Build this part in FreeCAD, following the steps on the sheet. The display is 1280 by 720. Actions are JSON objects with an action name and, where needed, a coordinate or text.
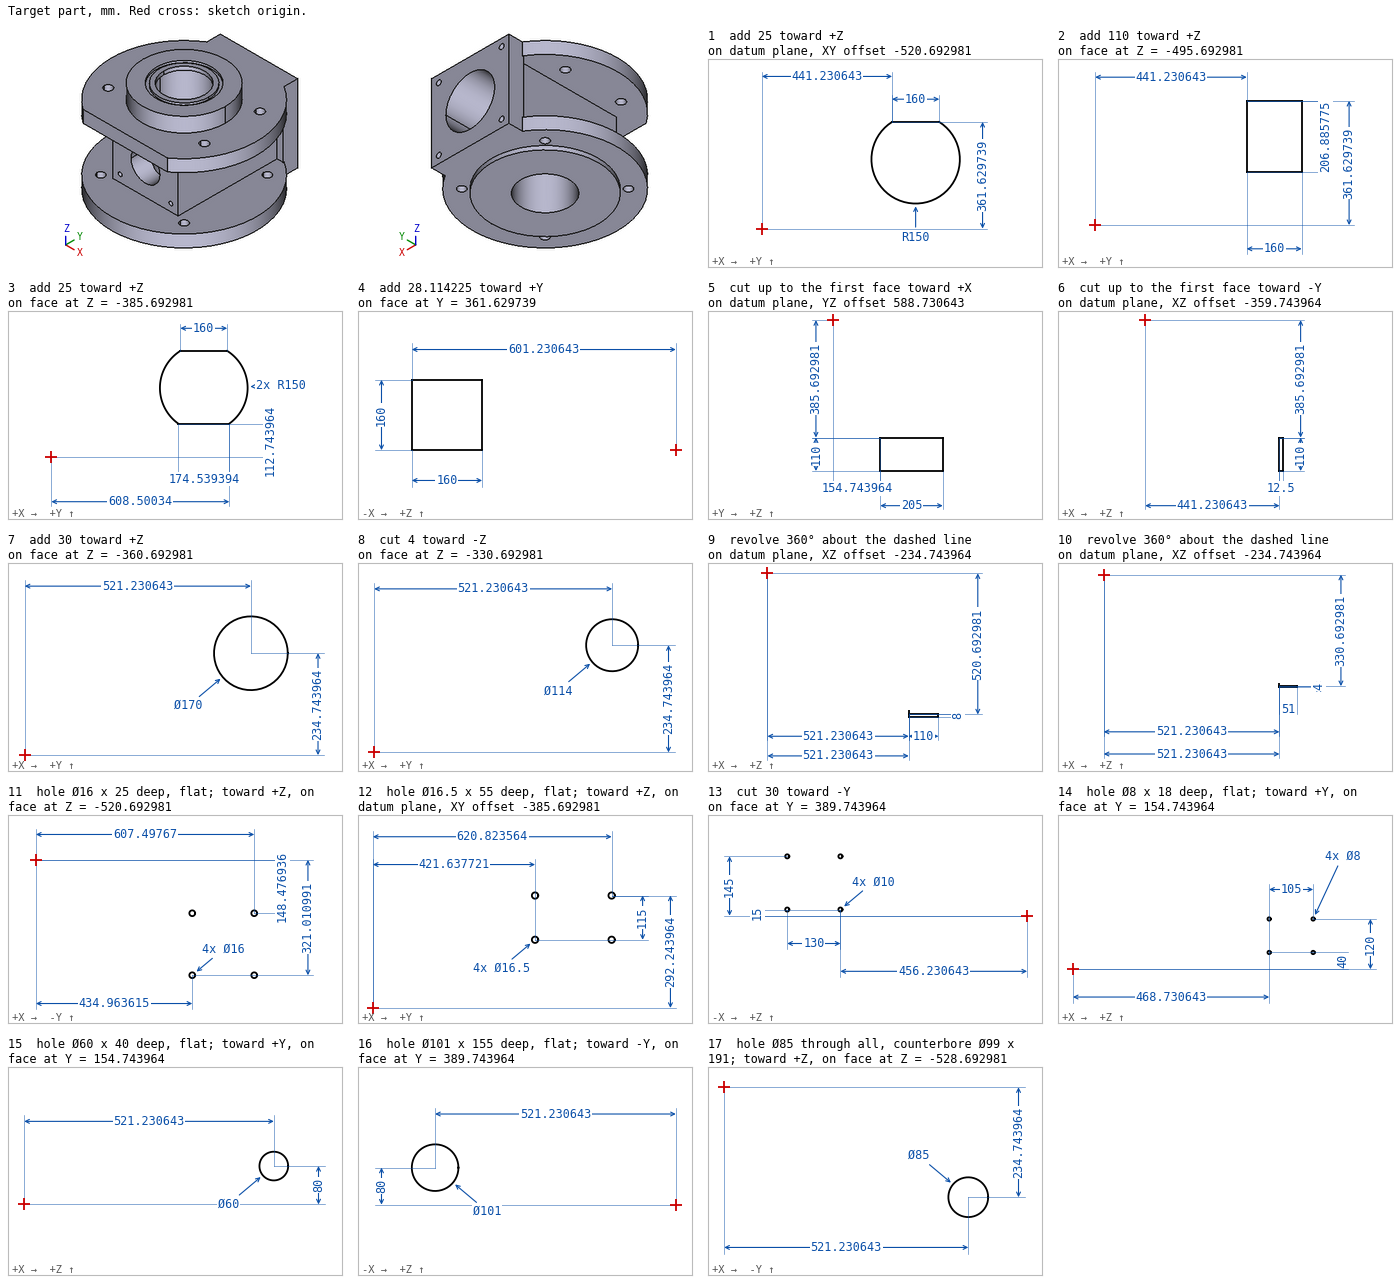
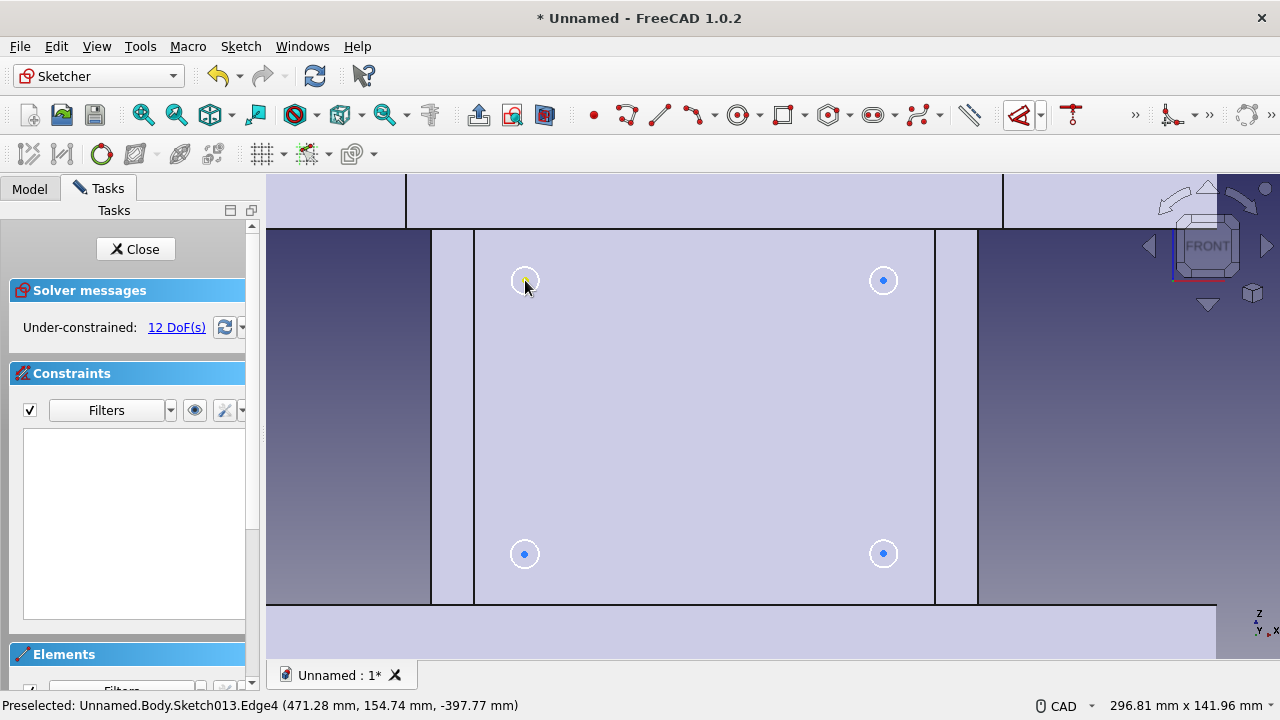
{"action": "left_click", "coordinate": [535, 544]}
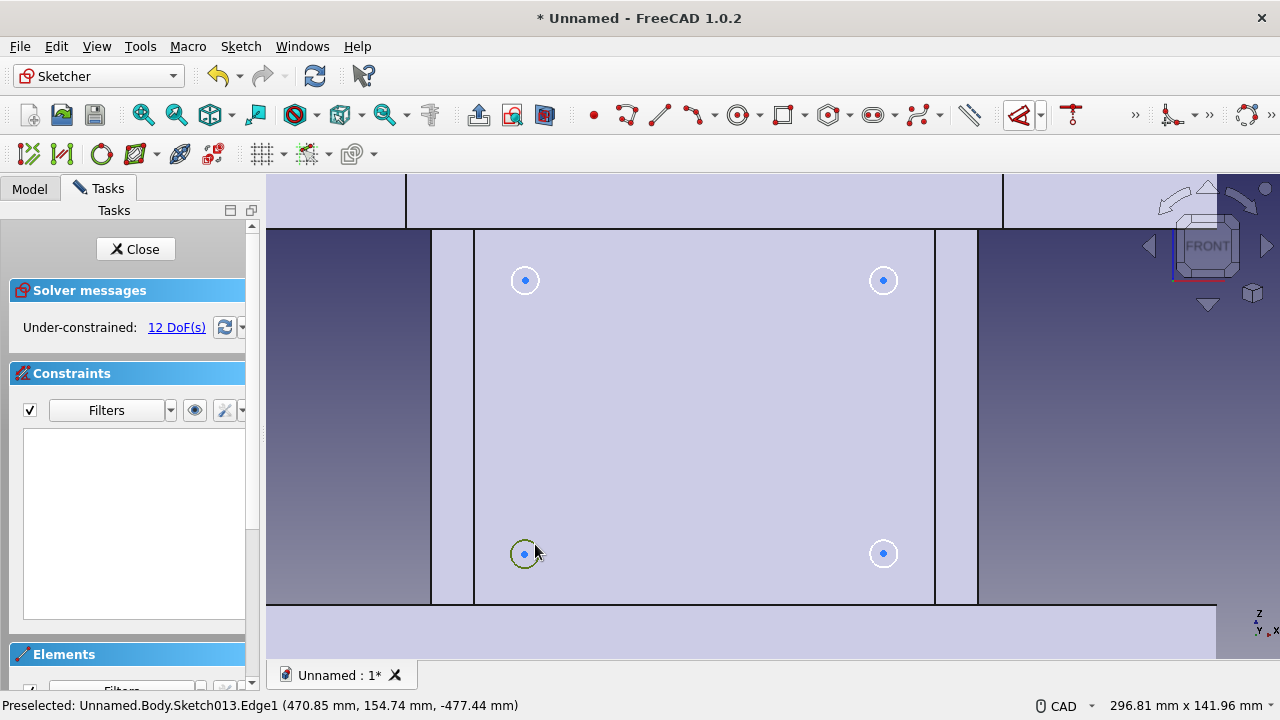
{"action": "left_click", "coordinate": [893, 271]}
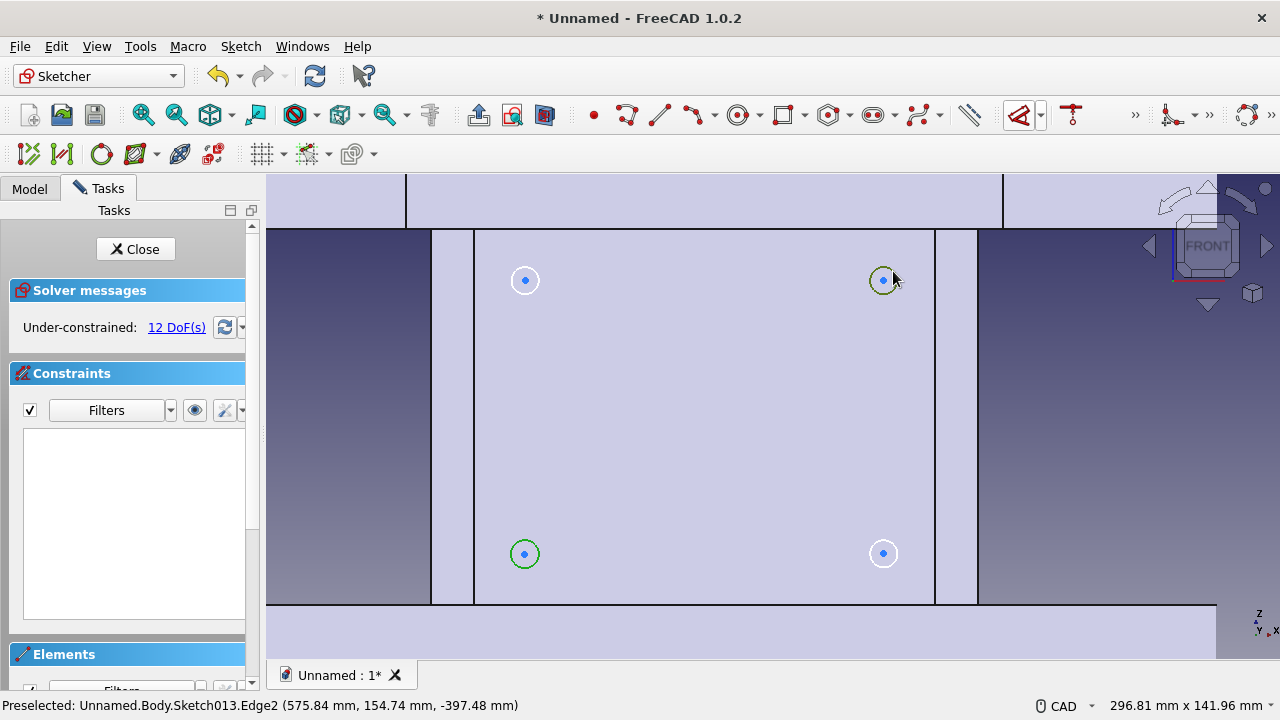
{"action": "left_click", "coordinate": [893, 544]}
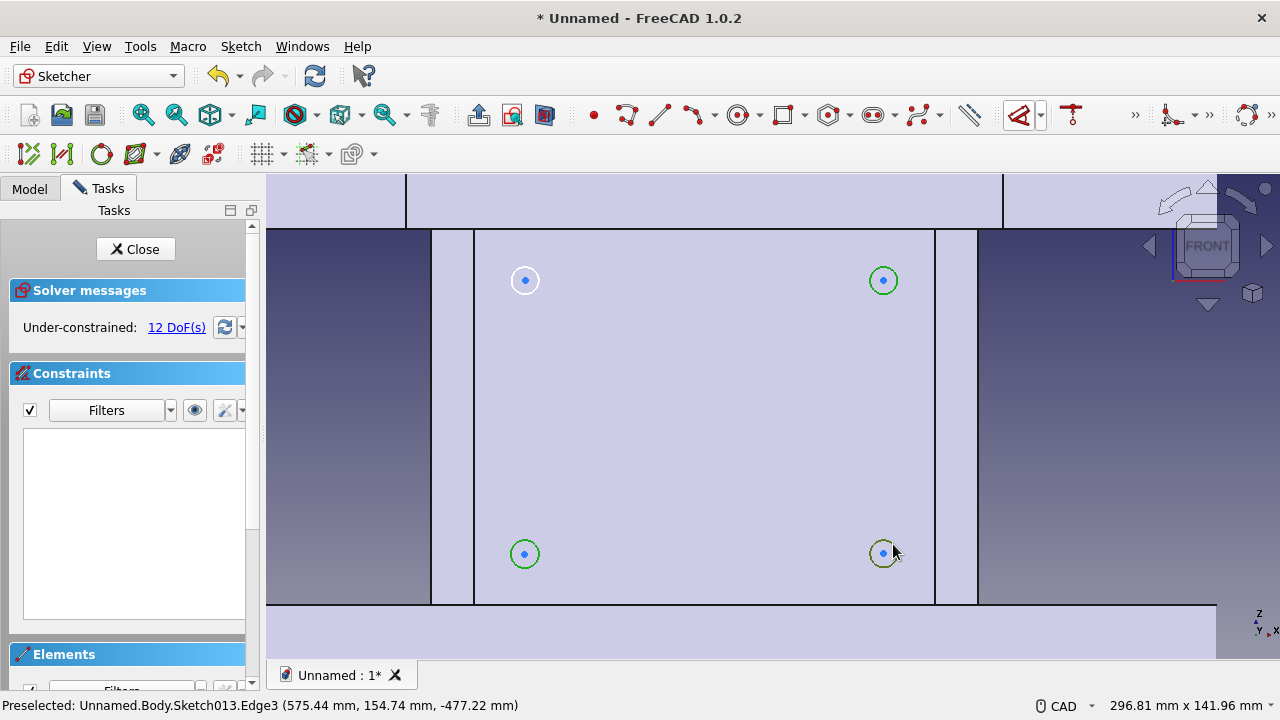
{"action": "left_click", "coordinate": [535, 271]}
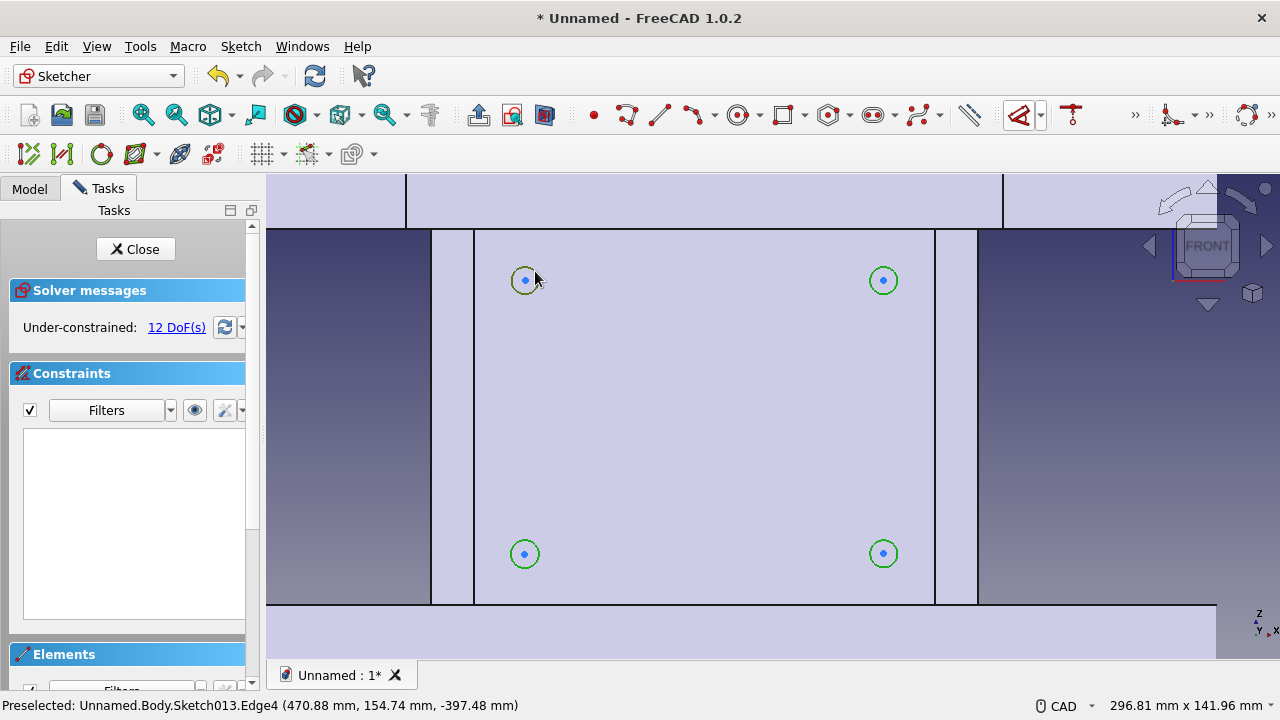
{"action": "key", "text": "e"}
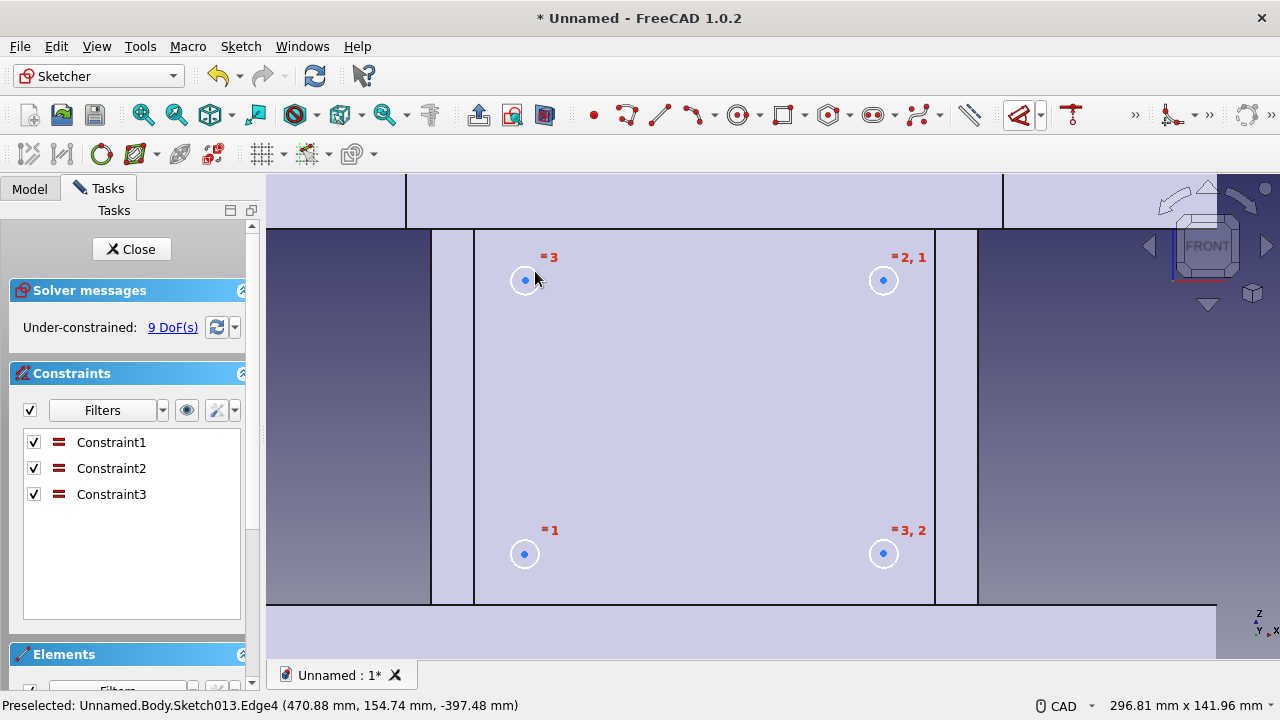
{"action": "left_click", "coordinate": [884, 281]}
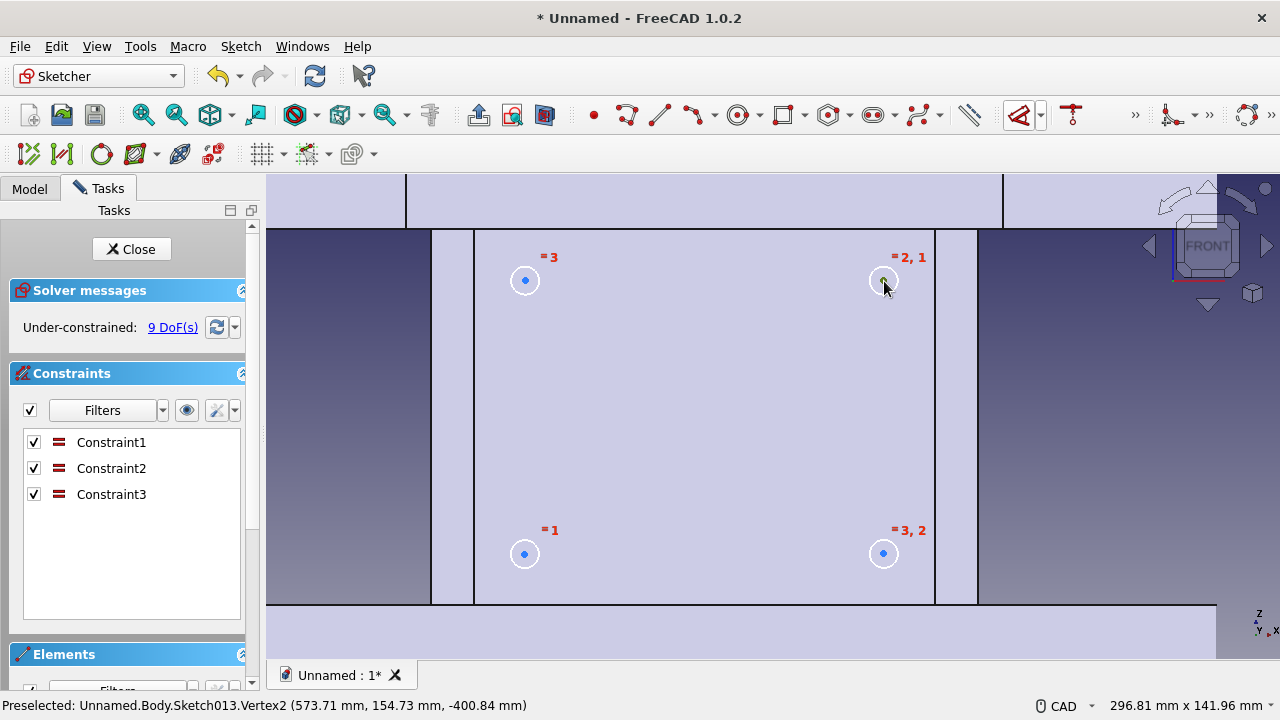
{"action": "left_click", "coordinate": [884, 554]}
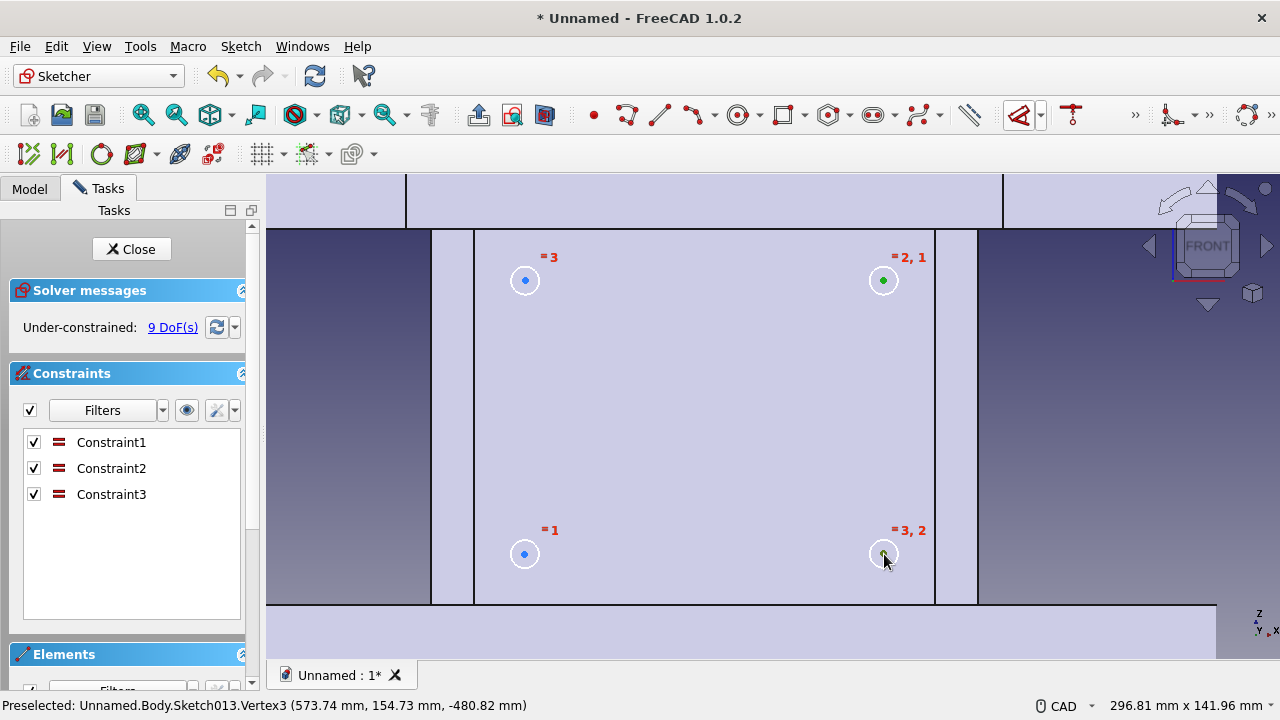
{"action": "key", "text": "v"}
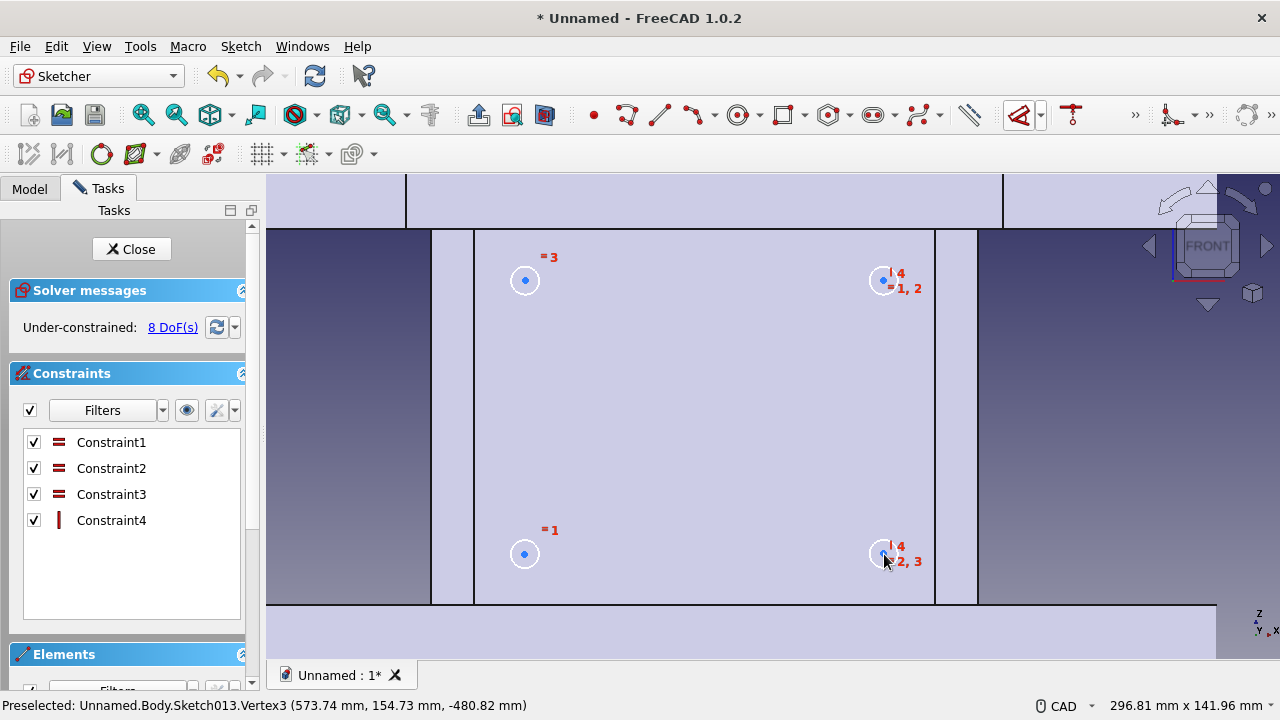
{"action": "left_click", "coordinate": [525, 554]}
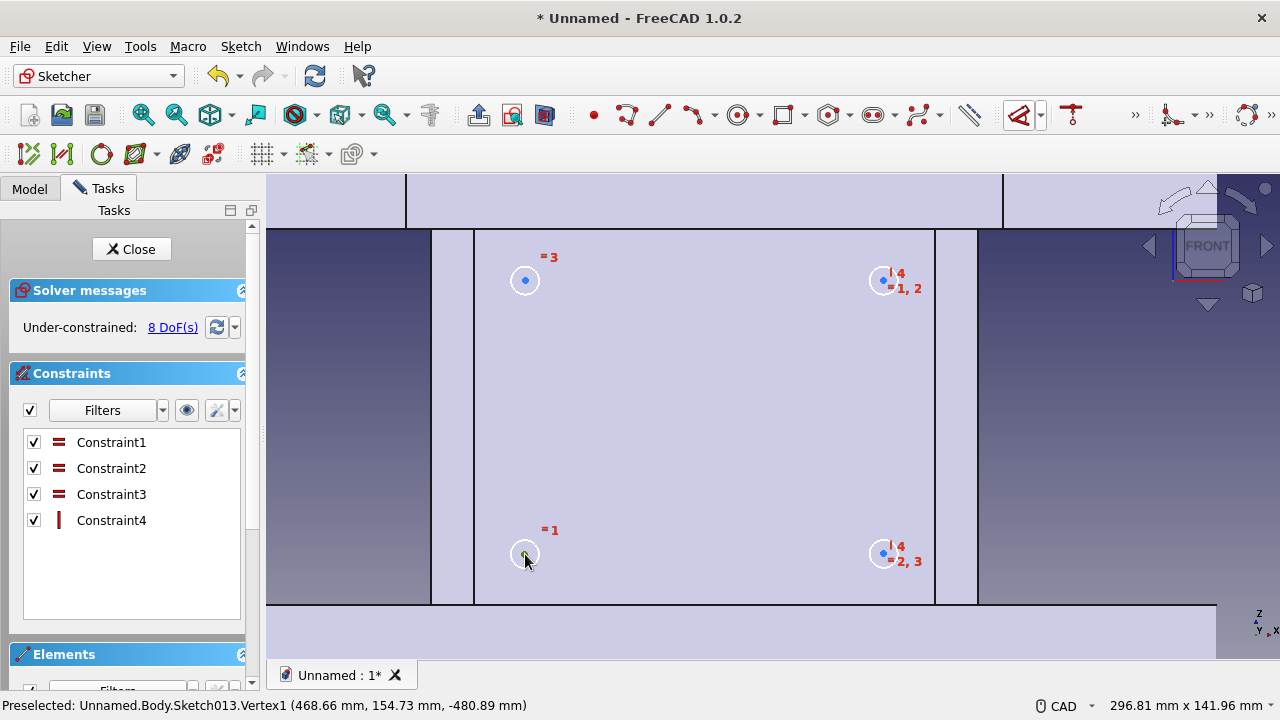
{"action": "left_click", "coordinate": [884, 554]}